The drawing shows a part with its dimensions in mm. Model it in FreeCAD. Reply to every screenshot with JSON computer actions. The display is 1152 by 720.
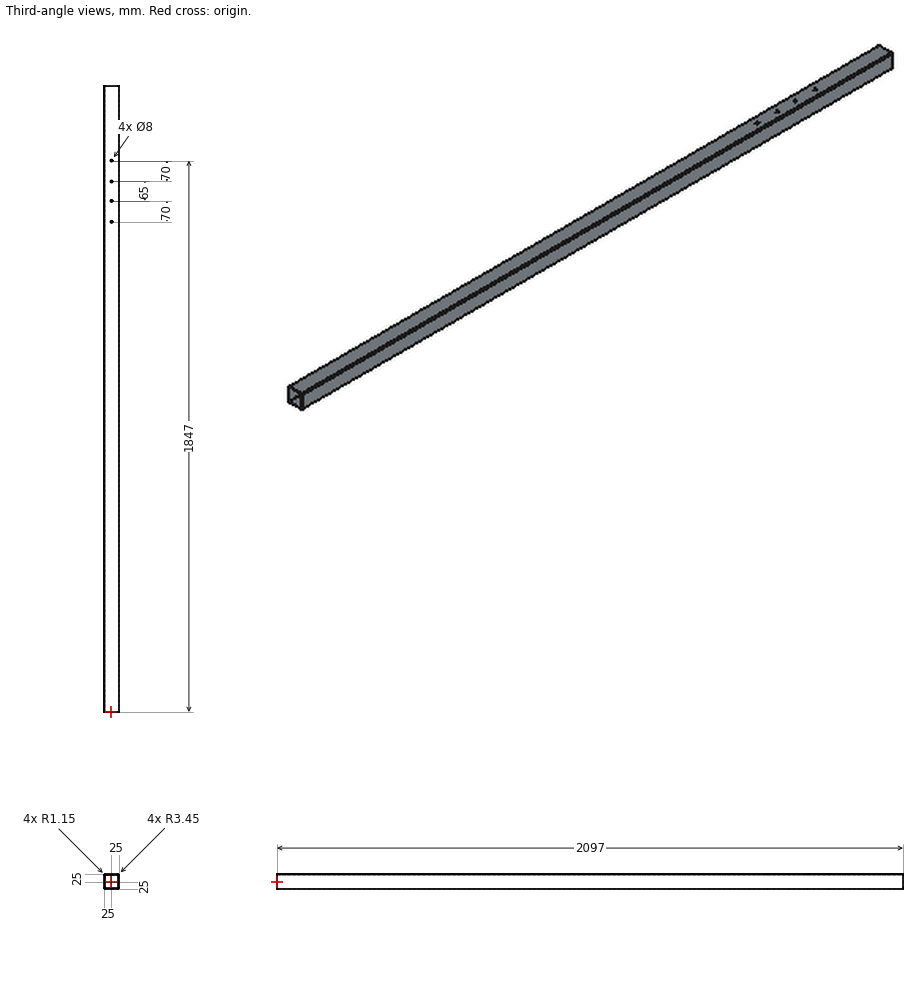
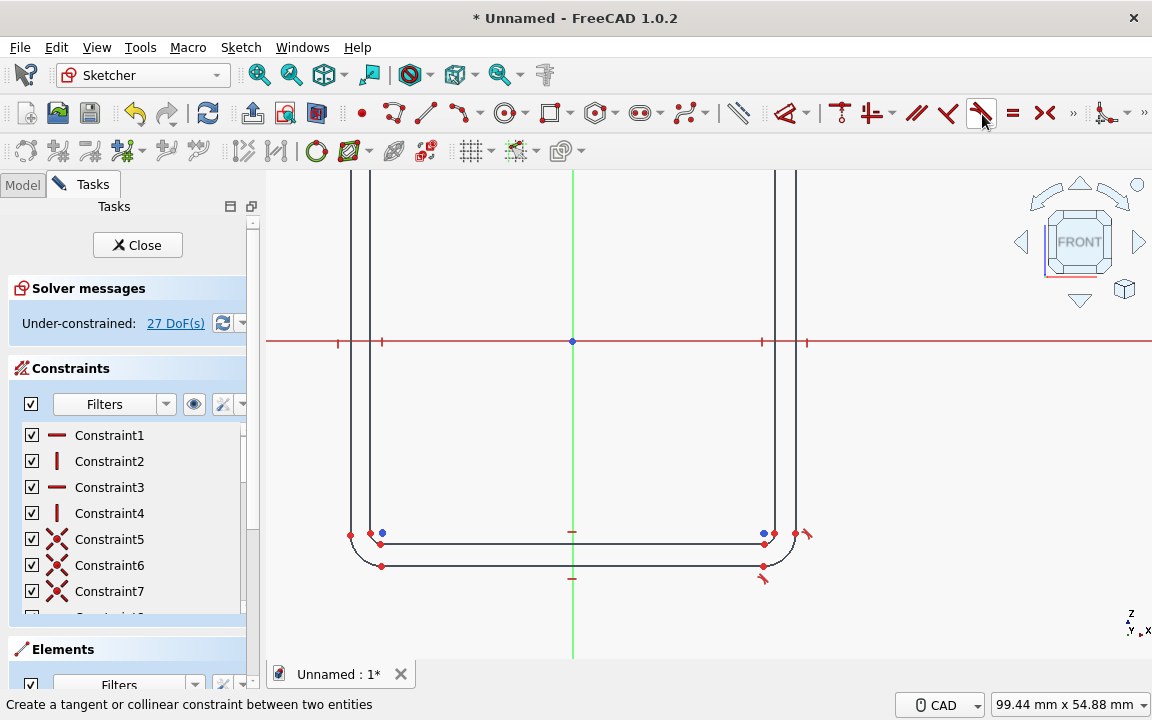
{"action": "left_click", "coordinate": [649, 566]}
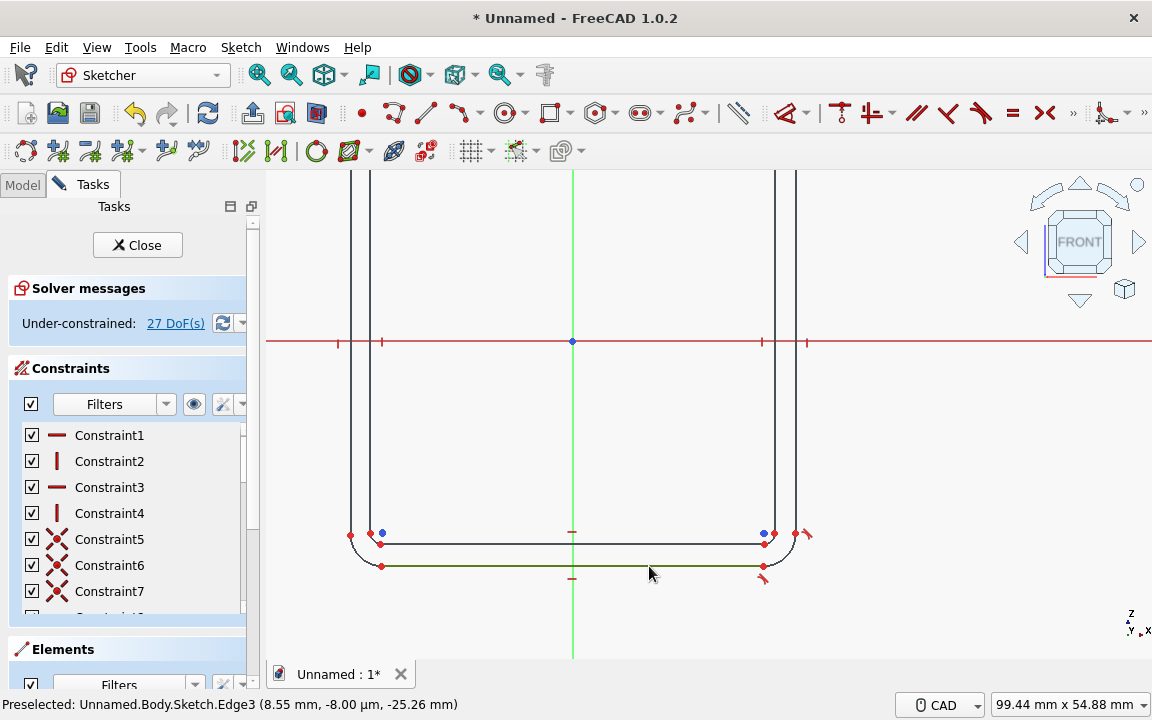
{"action": "left_click", "coordinate": [354, 549]}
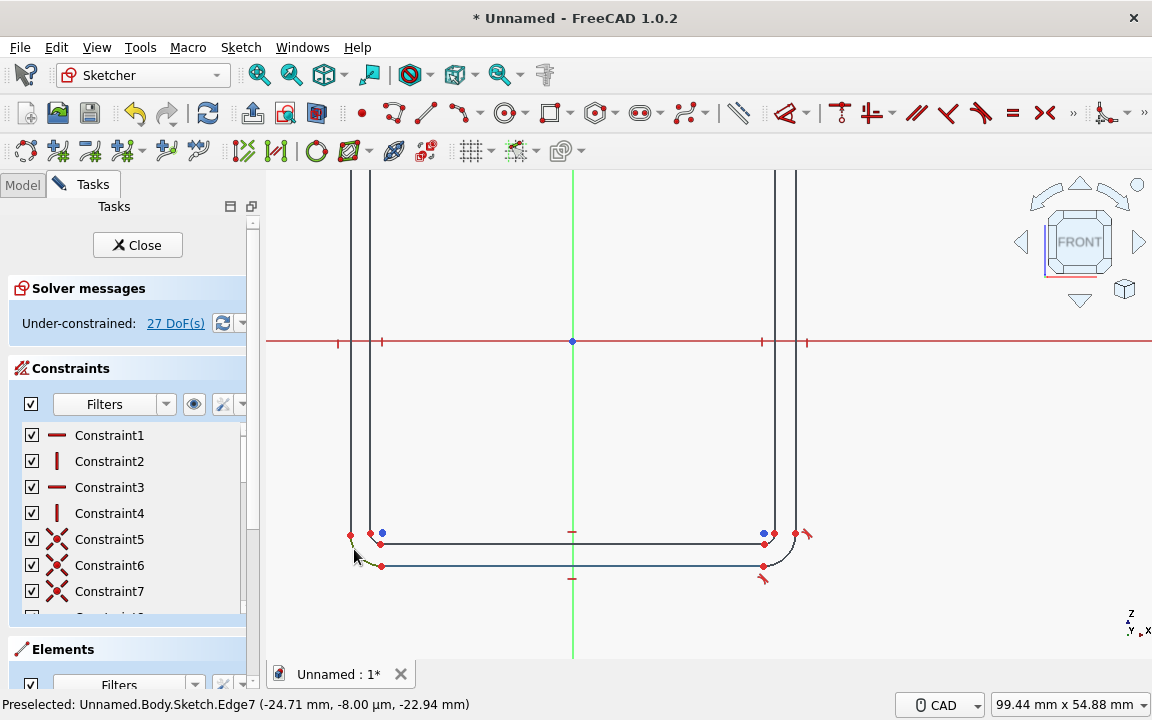
{"action": "left_click", "coordinate": [982, 114]}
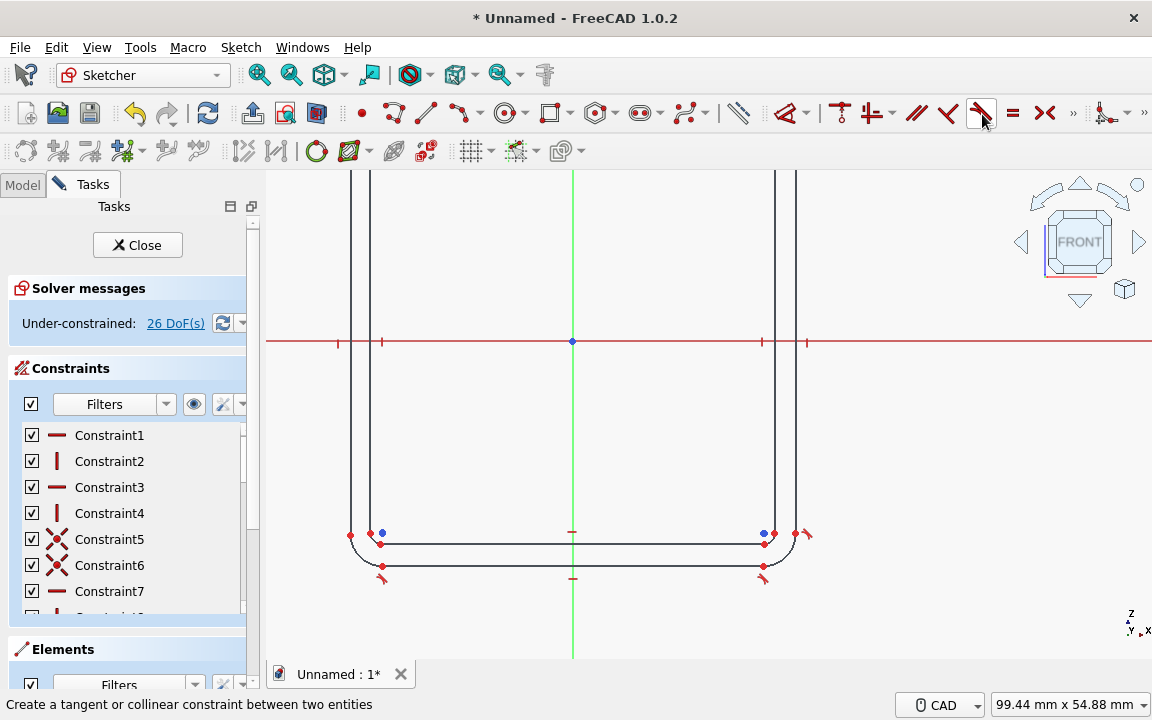
{"action": "left_click", "coordinate": [351, 420]}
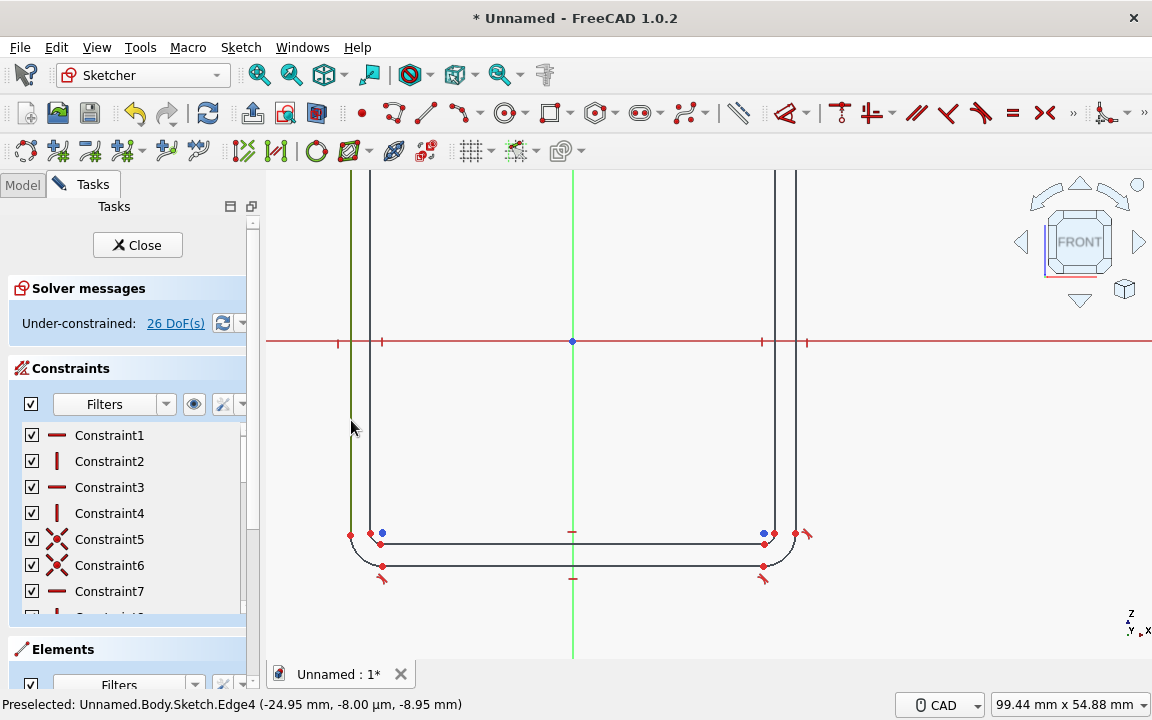
{"action": "left_click", "coordinate": [354, 549]}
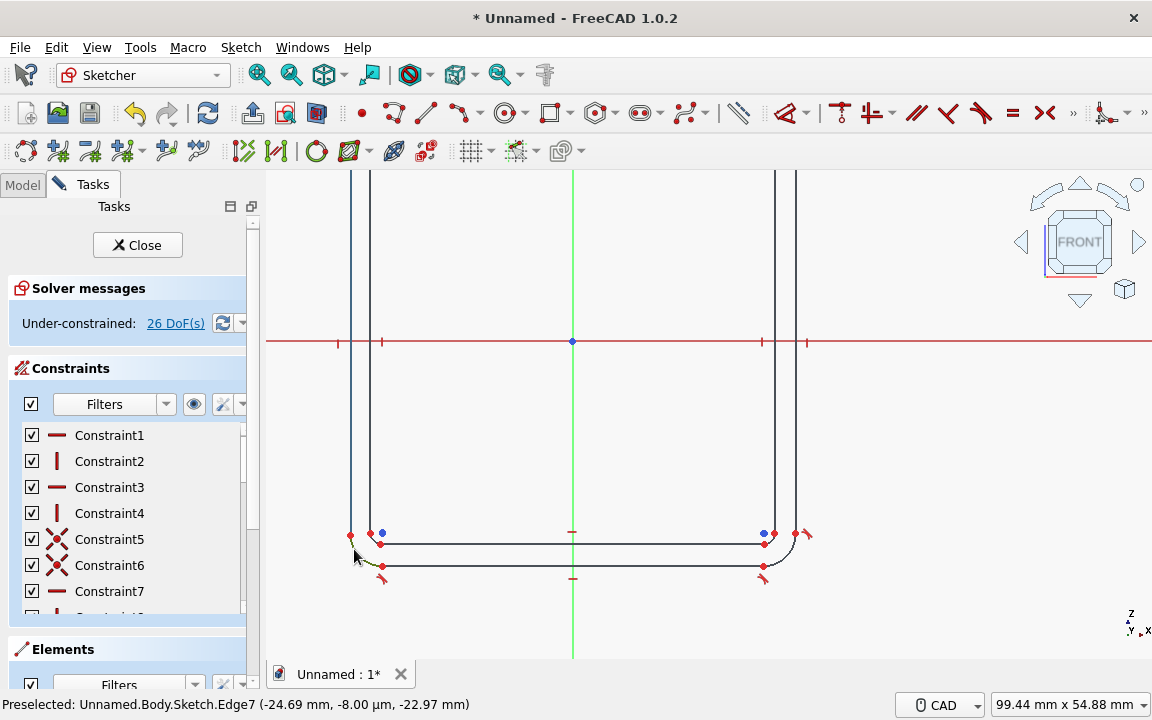
{"action": "left_click", "coordinate": [982, 114]}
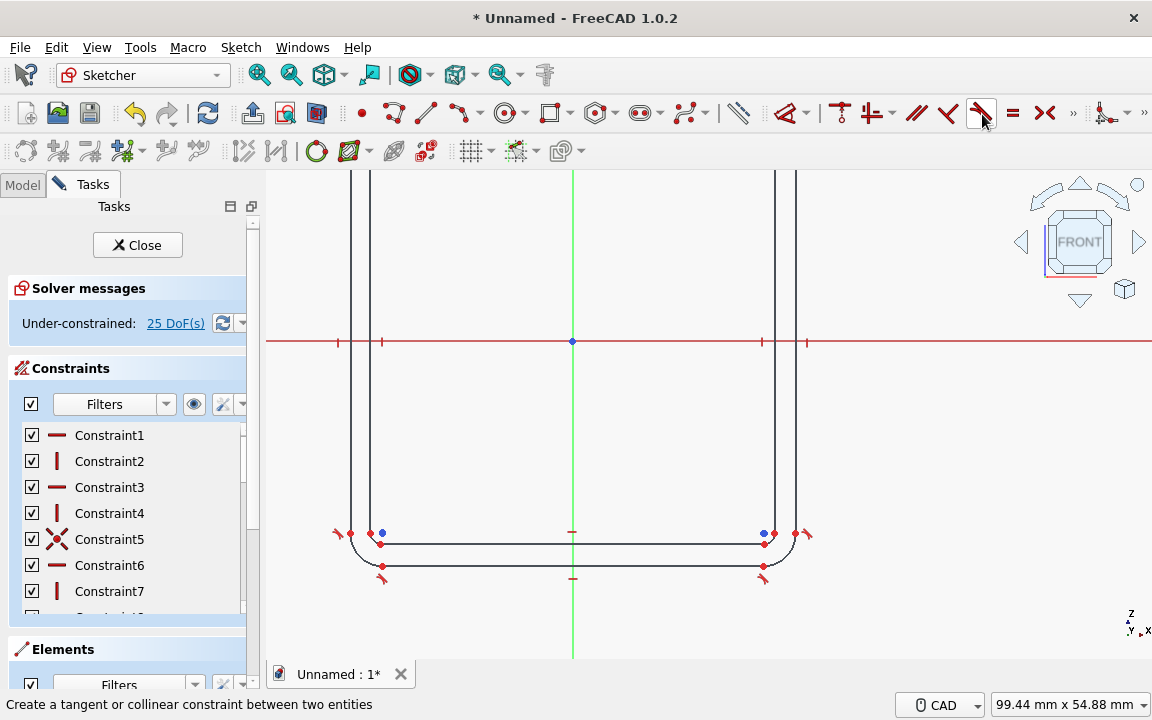
{"action": "left_click", "coordinate": [351, 419]}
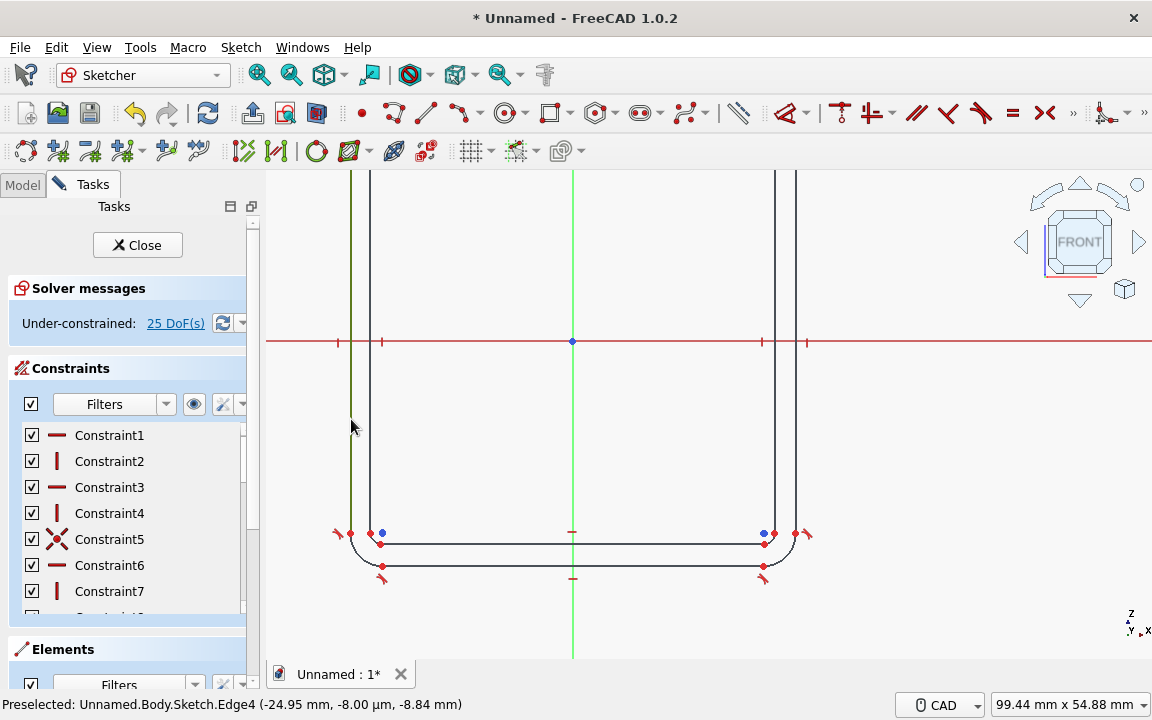
{"action": "scroll", "coordinate": [778, 563], "scroll_direction": "down", "scroll_amount": 2}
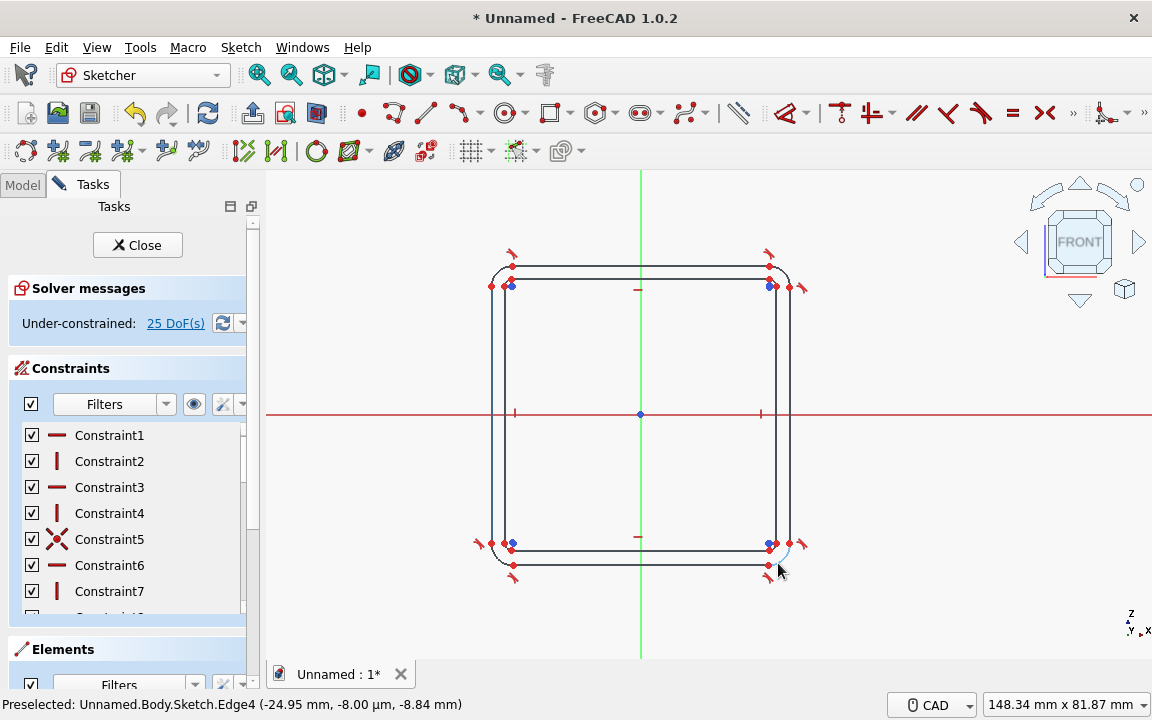
{"action": "scroll", "coordinate": [503, 268], "scroll_direction": "up", "scroll_amount": 2}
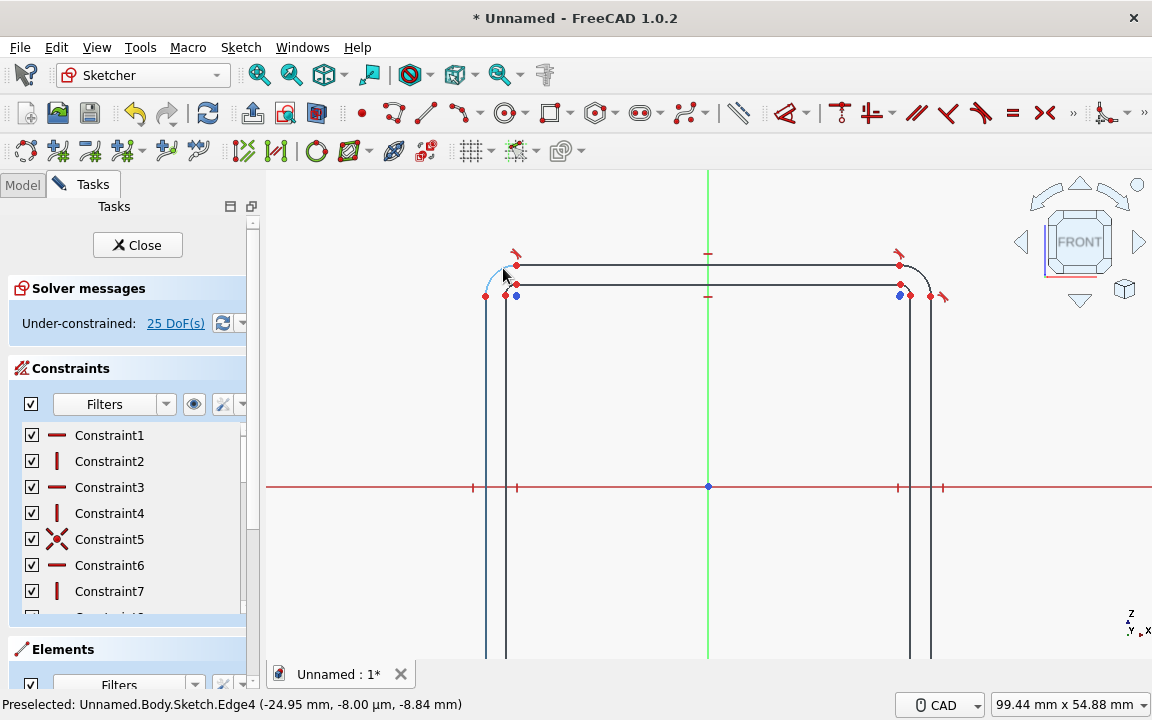
{"action": "left_click", "coordinate": [503, 269]}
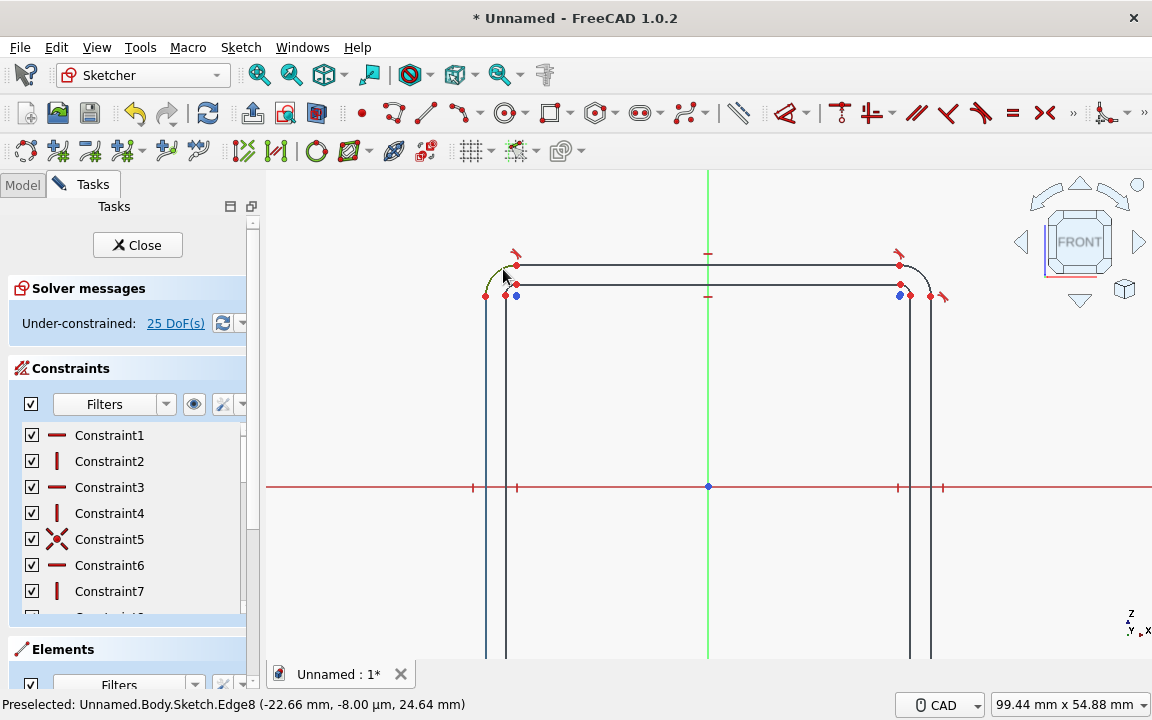
{"action": "left_click", "coordinate": [982, 114]}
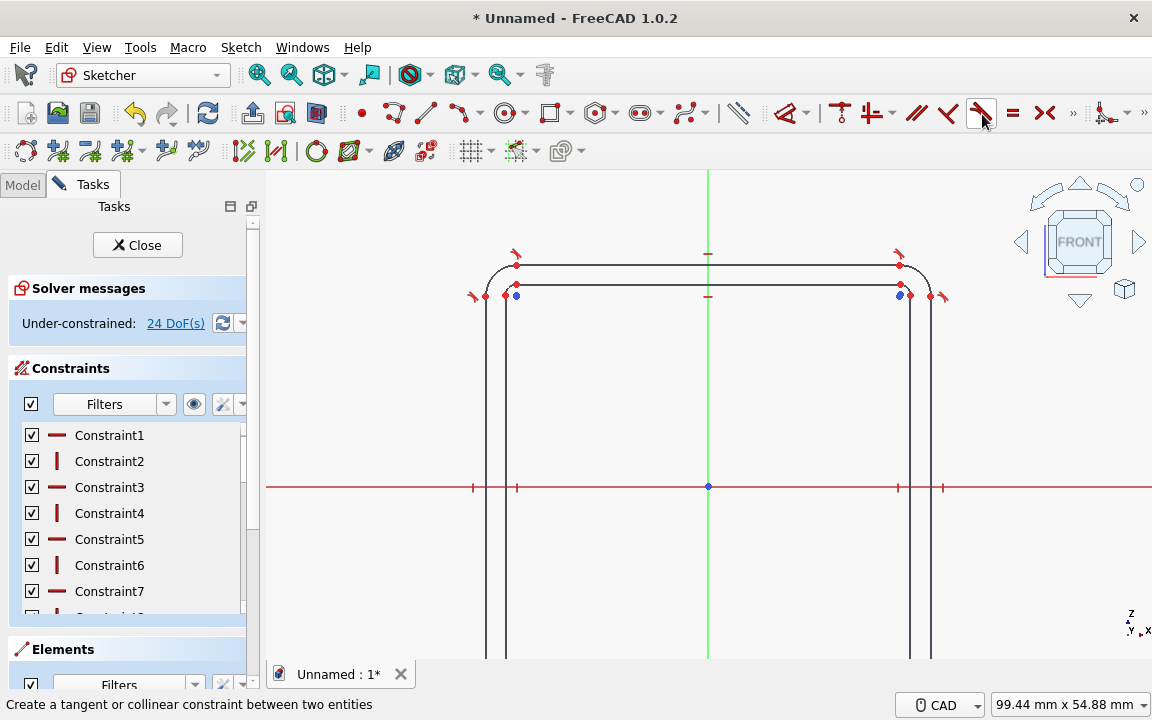
{"action": "left_click", "coordinate": [785, 285]}